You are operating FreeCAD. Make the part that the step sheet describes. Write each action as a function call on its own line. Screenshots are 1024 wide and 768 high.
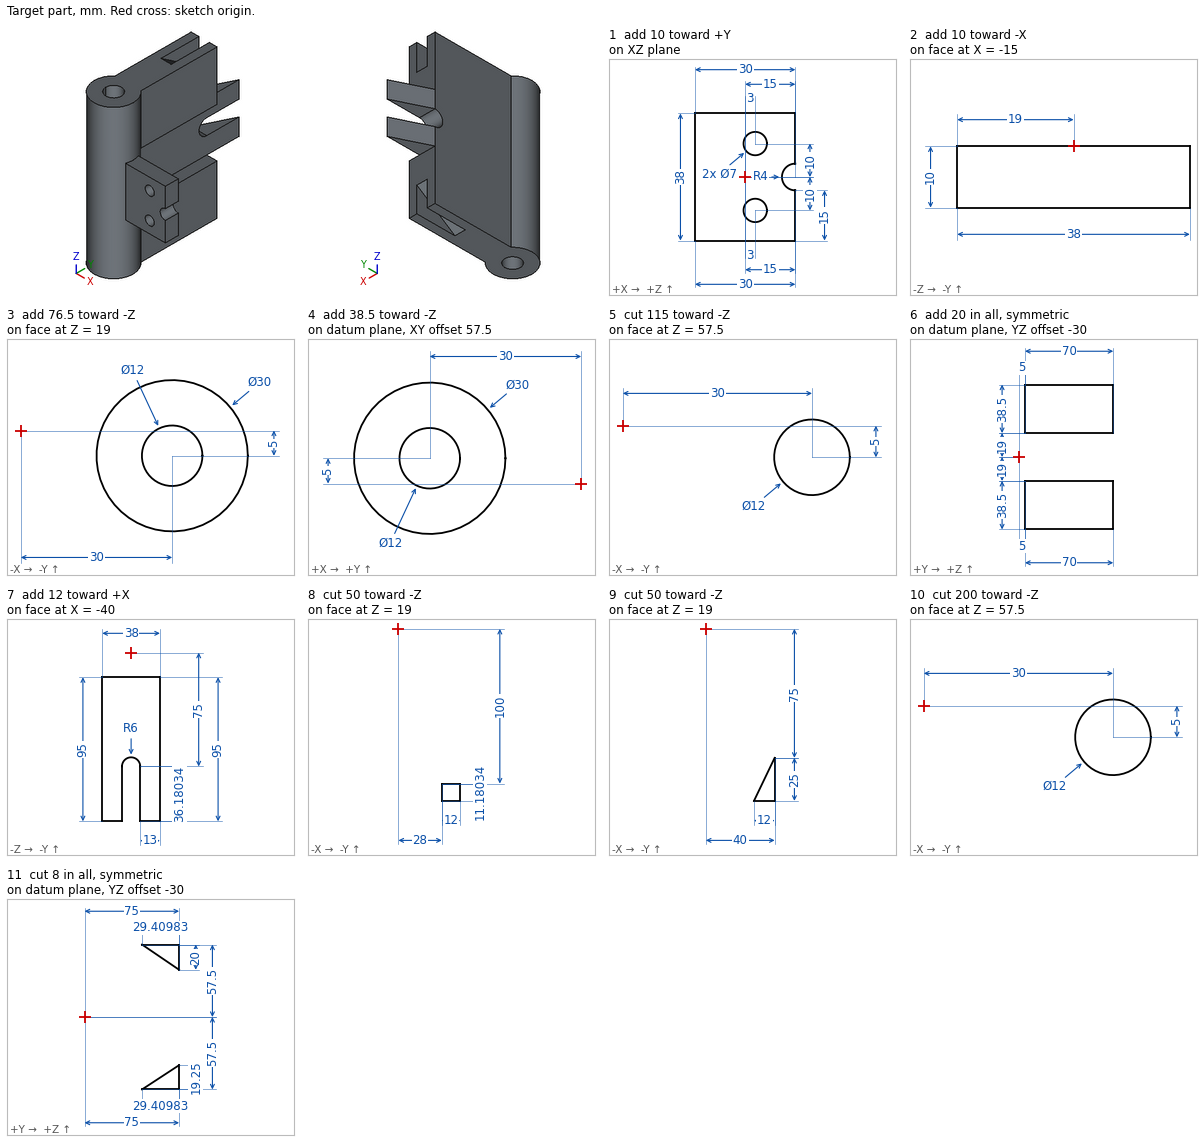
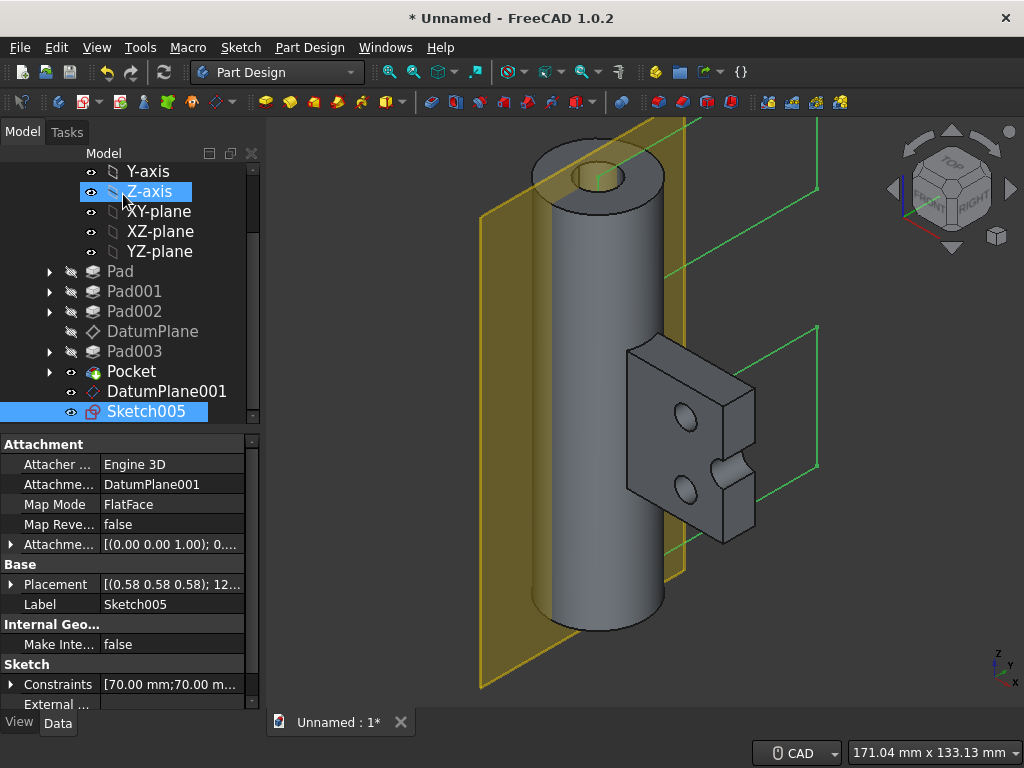
click(266, 102)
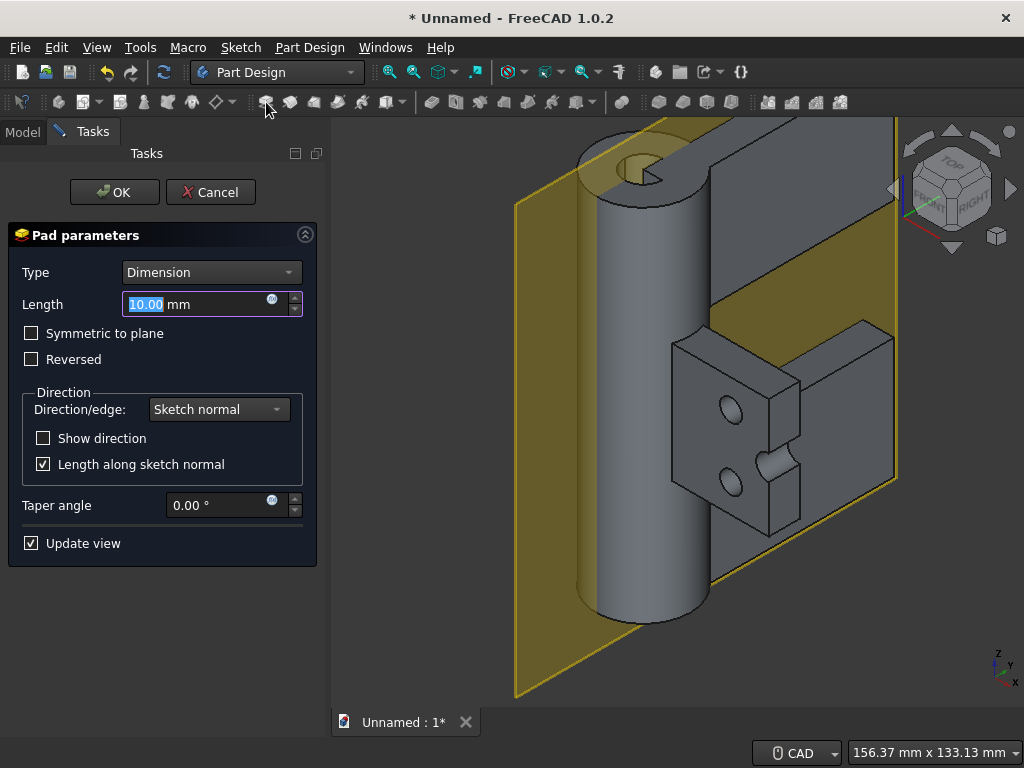
text(20)
key(Tab)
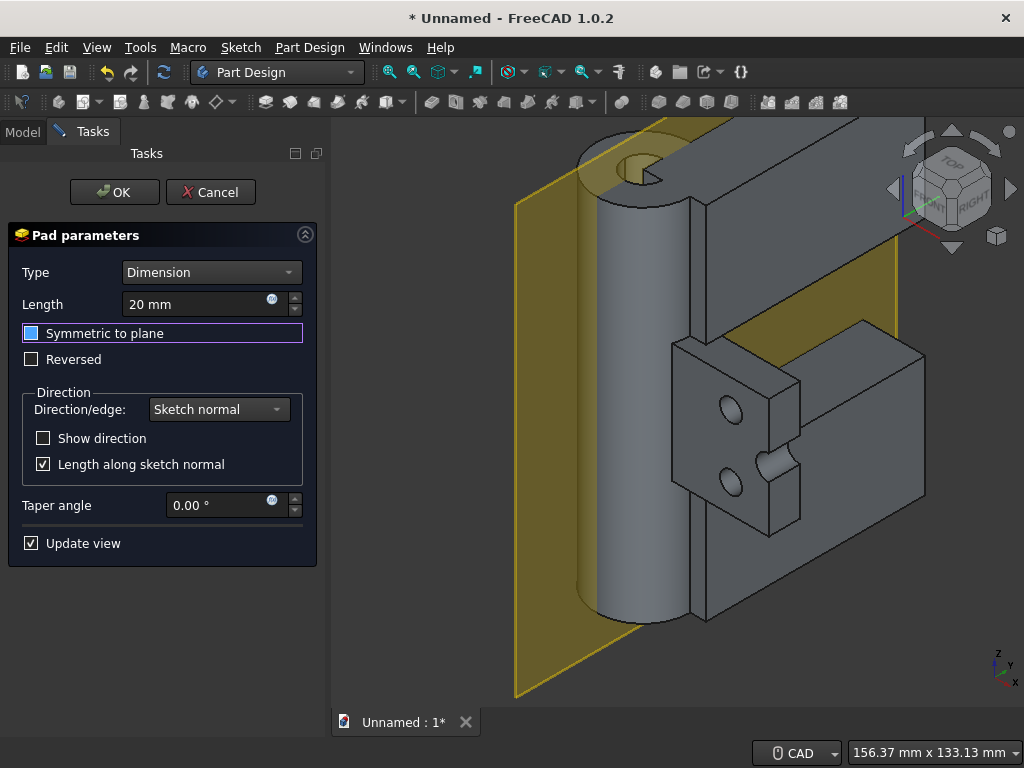
click(30, 333)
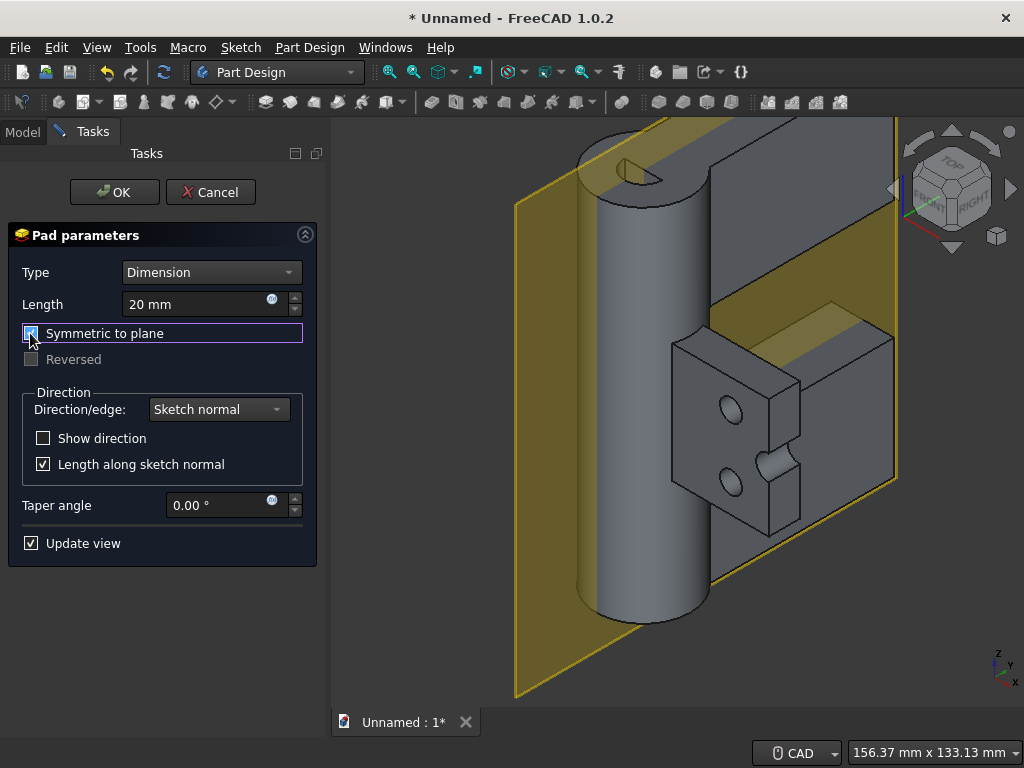
click(115, 192)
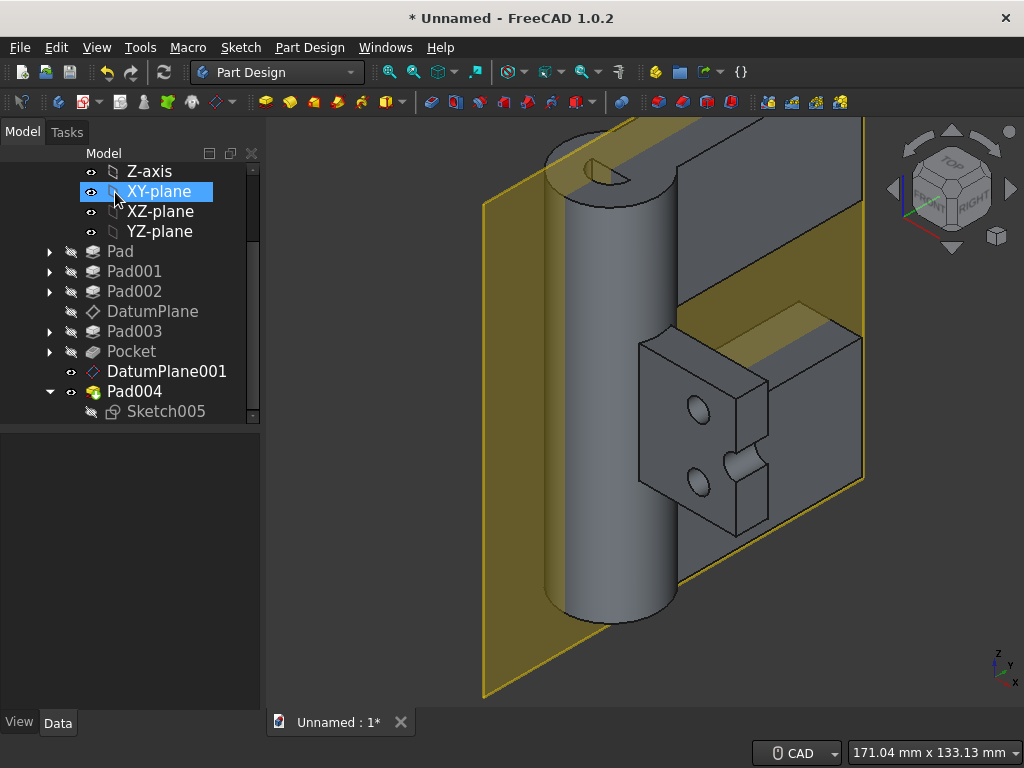
click(116, 372)
key(space)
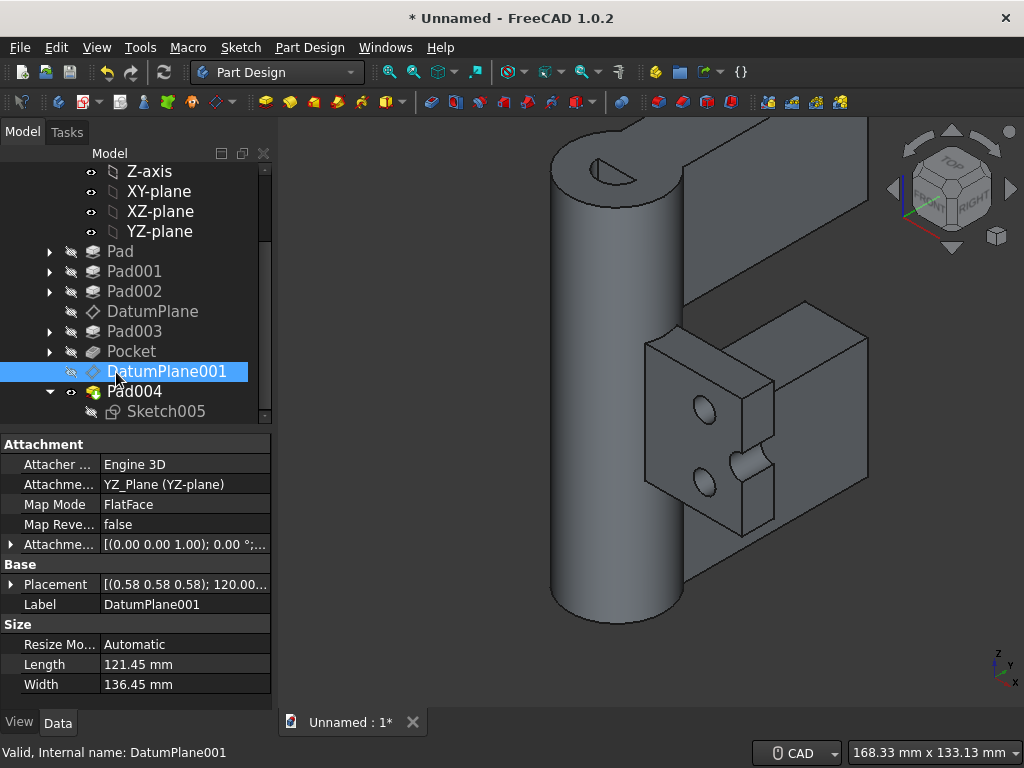
click(390, 72)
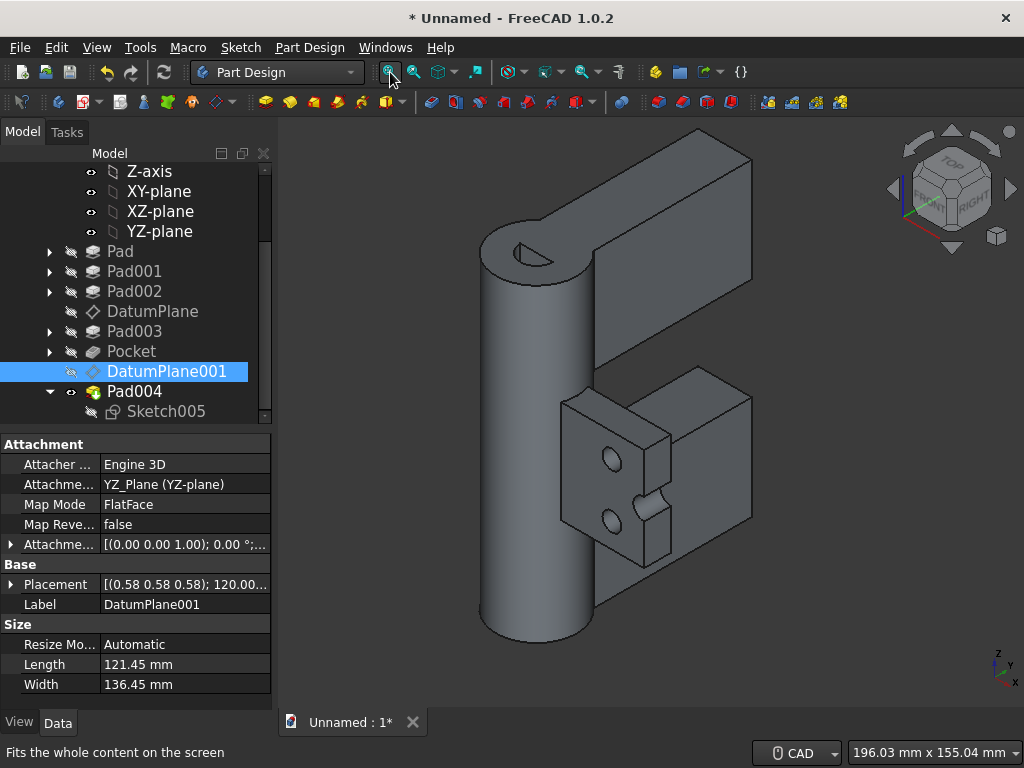
key(6)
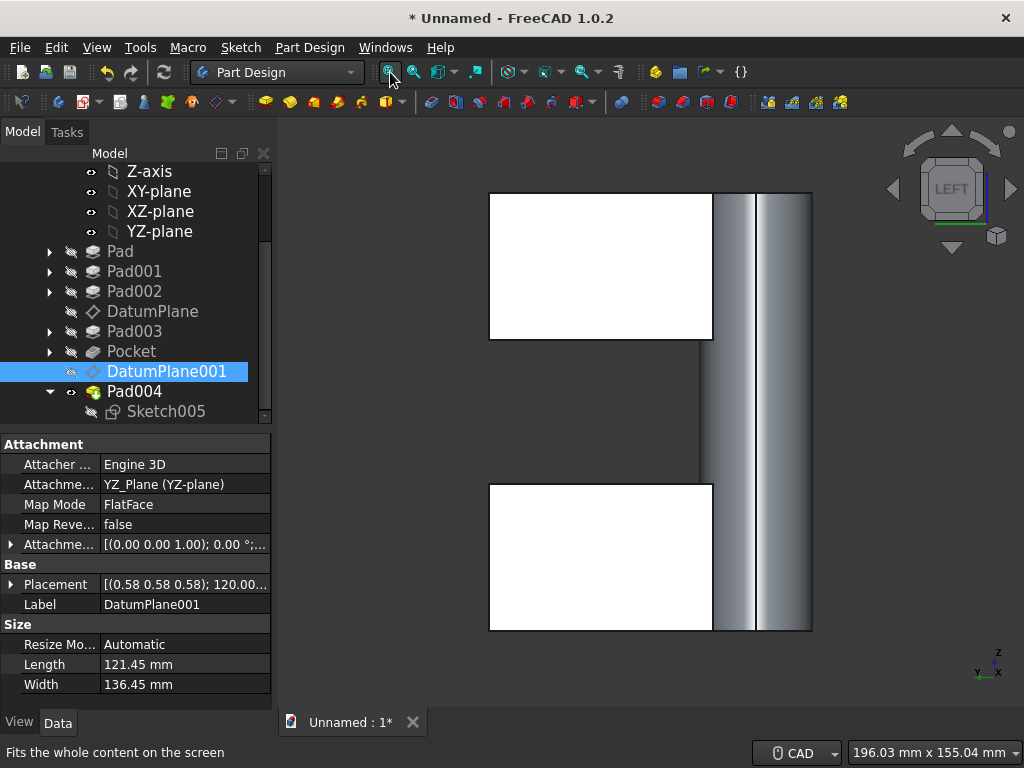
click(569, 265)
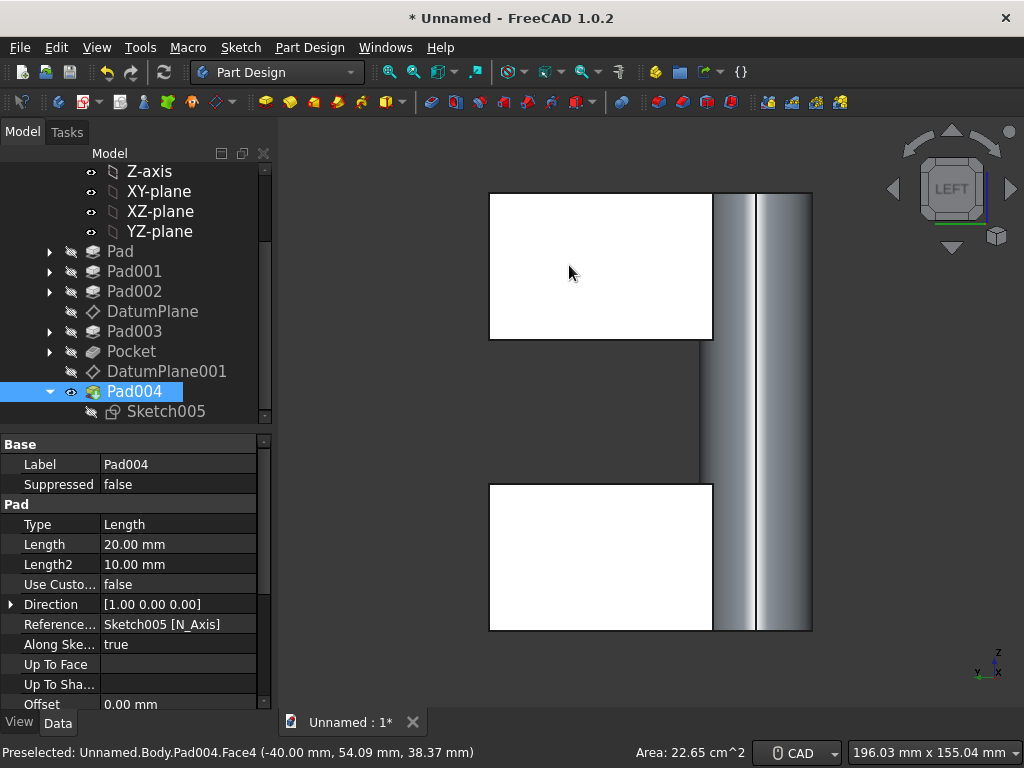
click(84, 102)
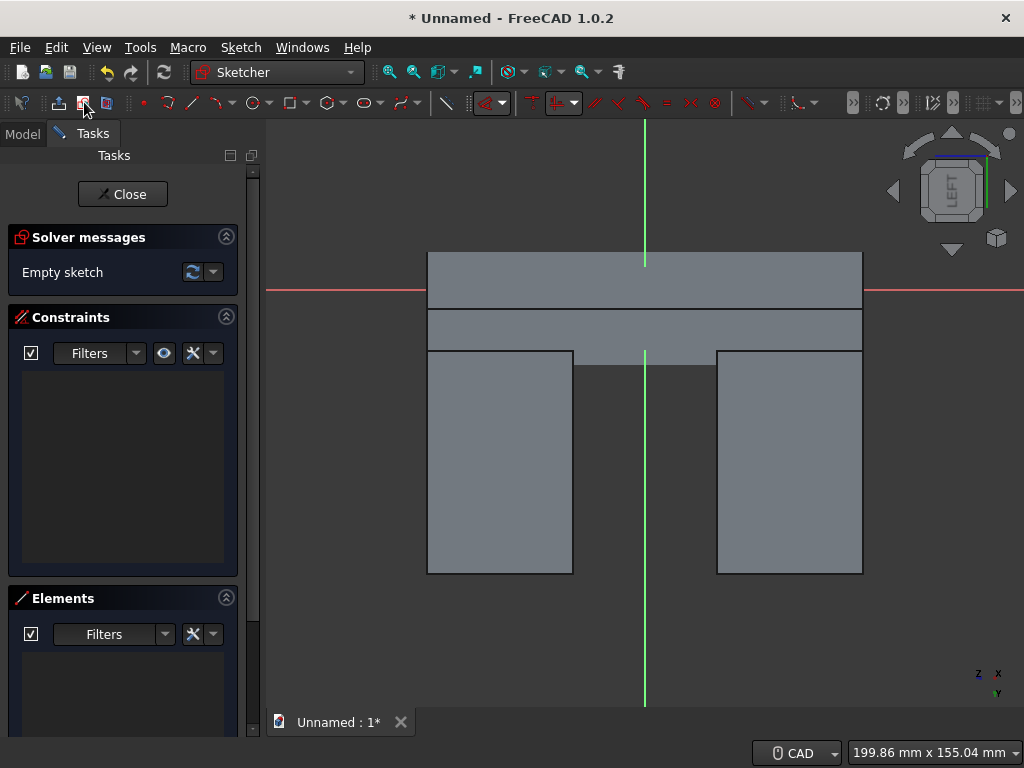
key(q)
key(s)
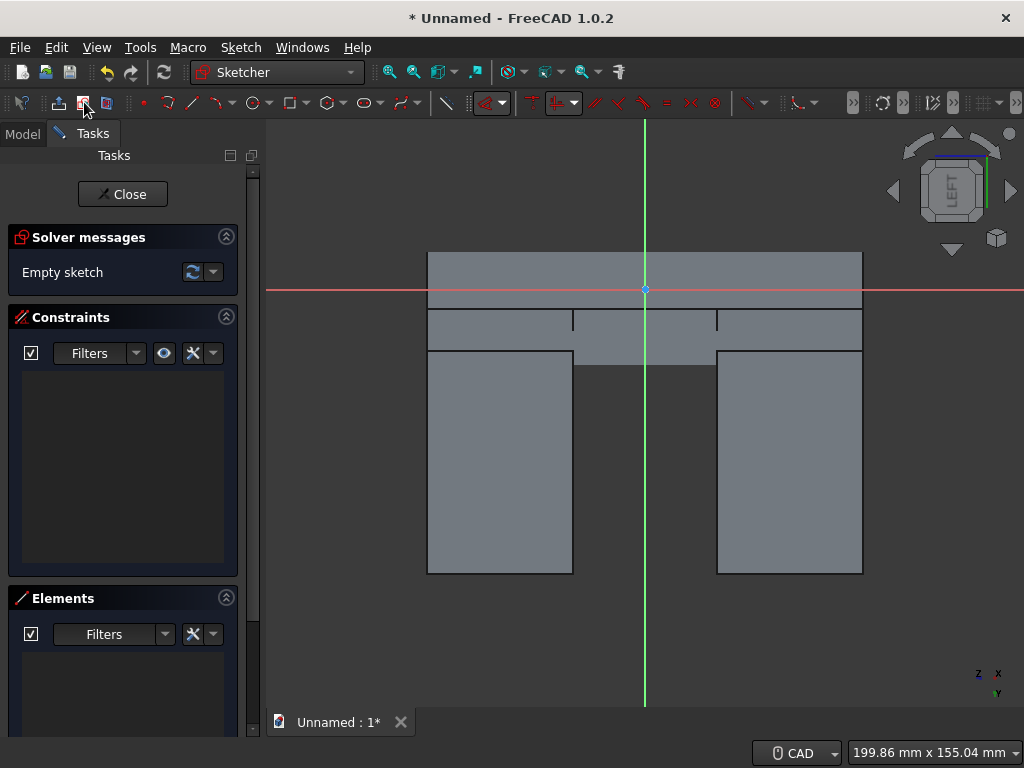
scroll(294, 147, down, 1)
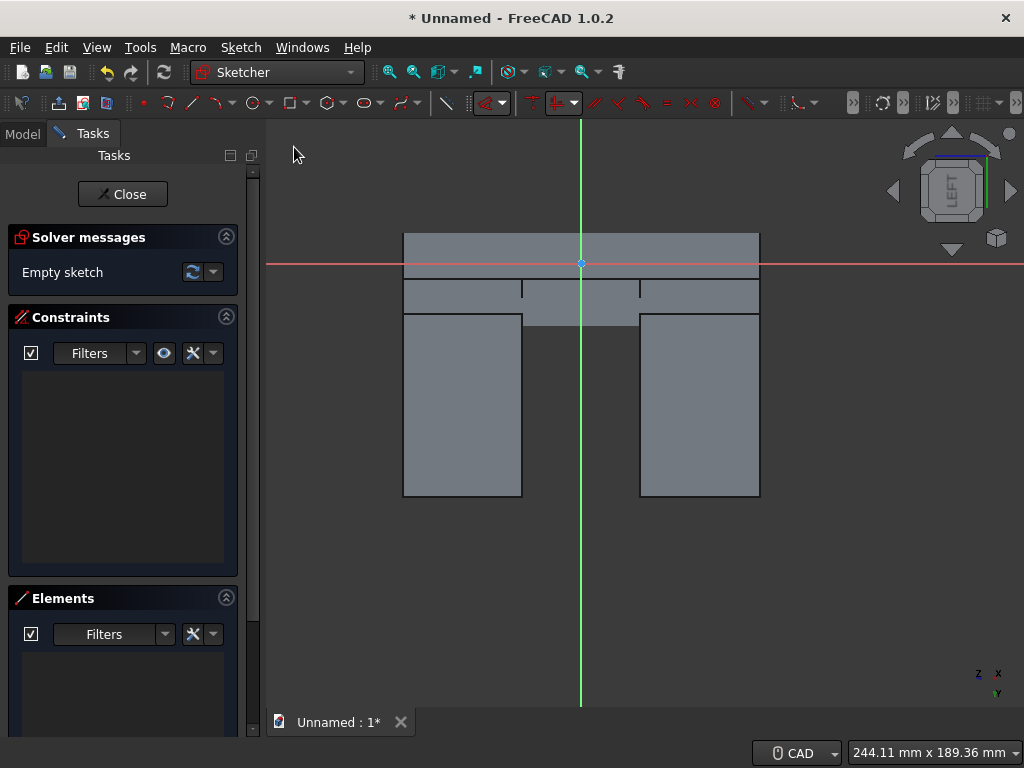
key(g)
key(m)